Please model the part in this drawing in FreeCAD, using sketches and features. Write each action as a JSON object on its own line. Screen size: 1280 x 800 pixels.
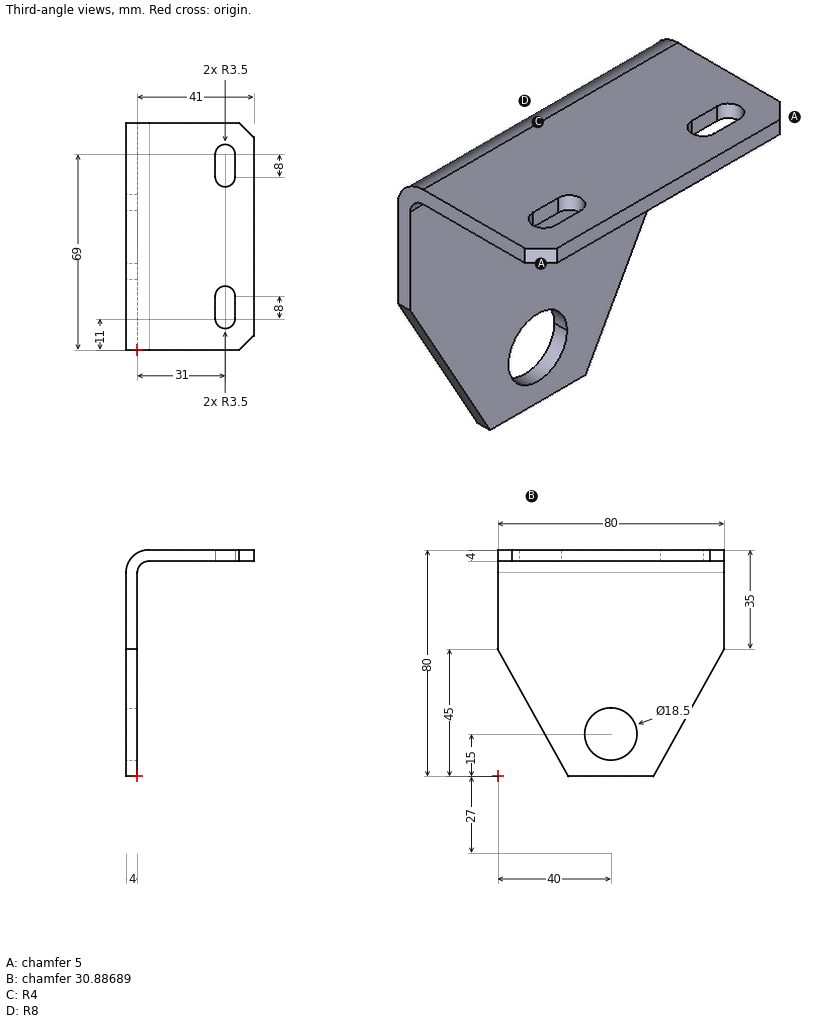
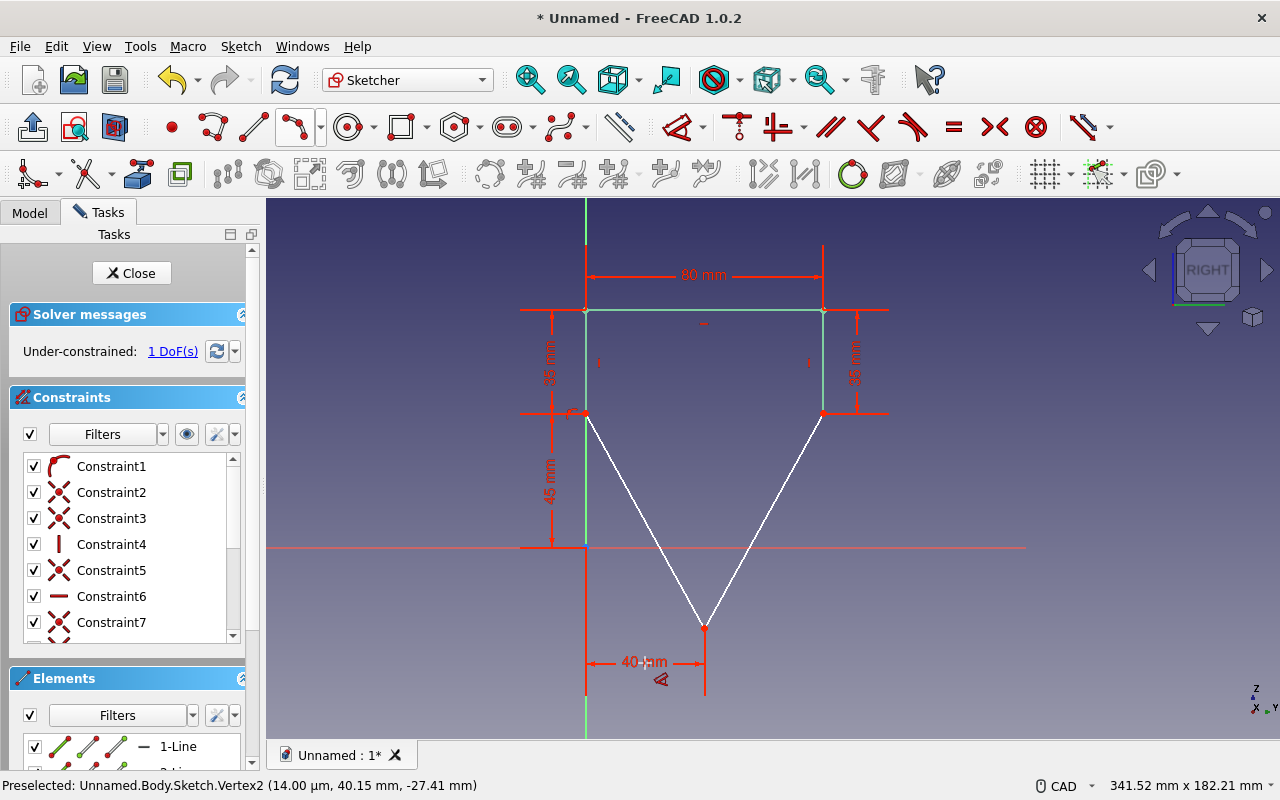
{"action": "left_click", "coordinate": [705, 629]}
{"action": "left_click", "coordinate": [552, 588]}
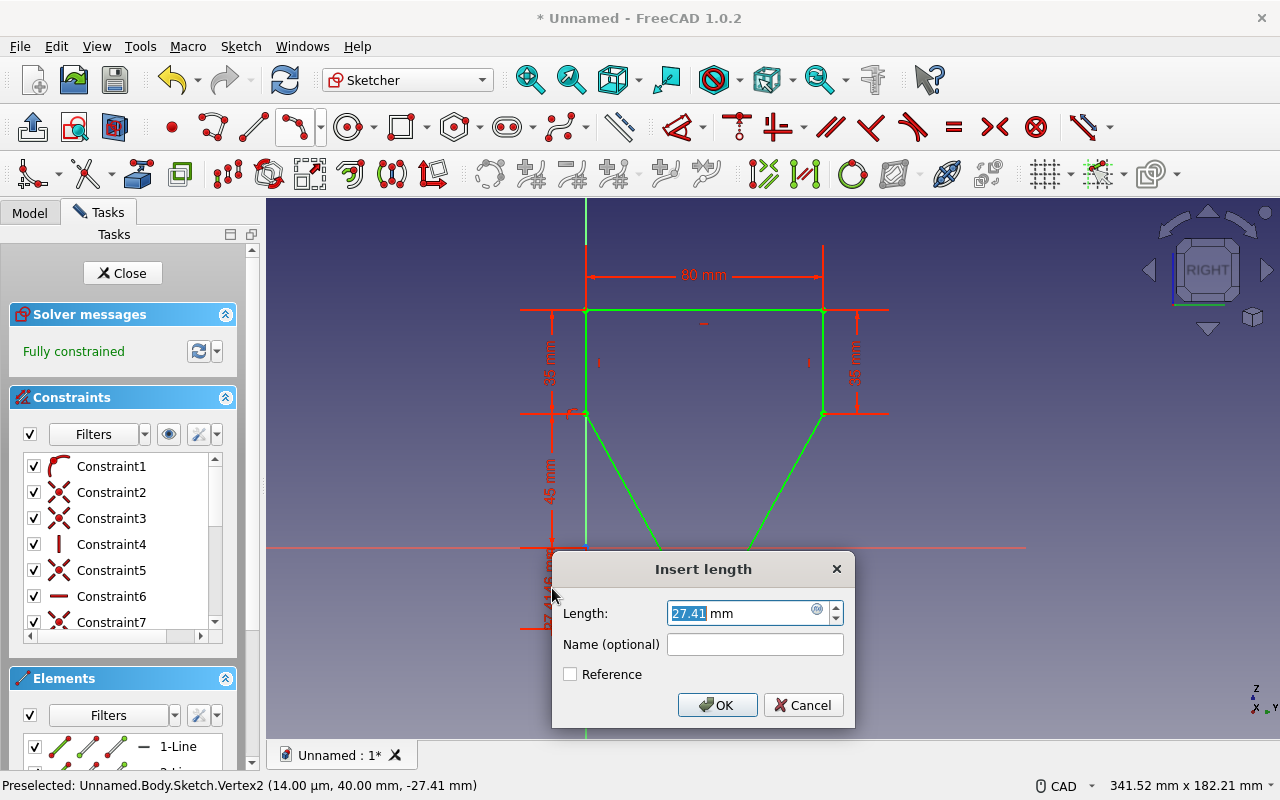
{"action": "type", "text": "27"}
{"action": "key", "text": "Return"}
{"action": "key", "text": "Escape"}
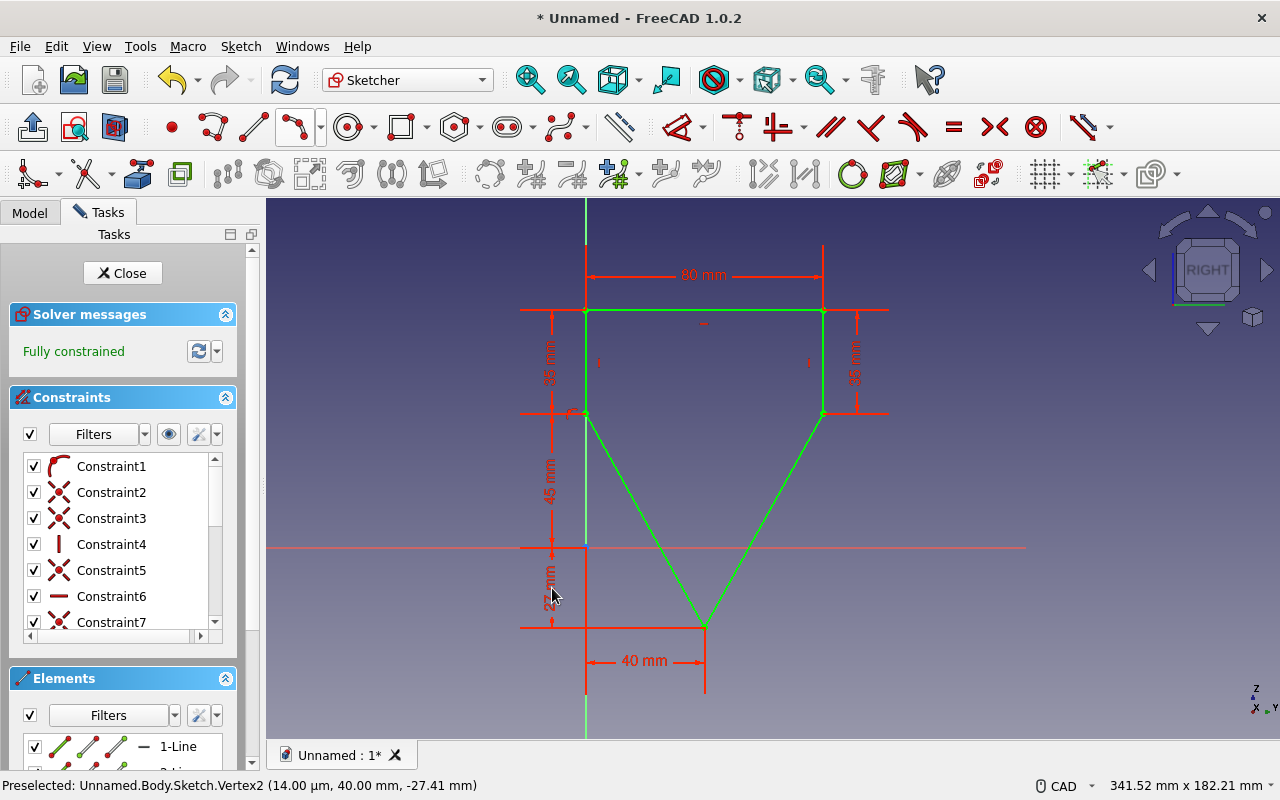
{"action": "left_click", "coordinate": [123, 273]}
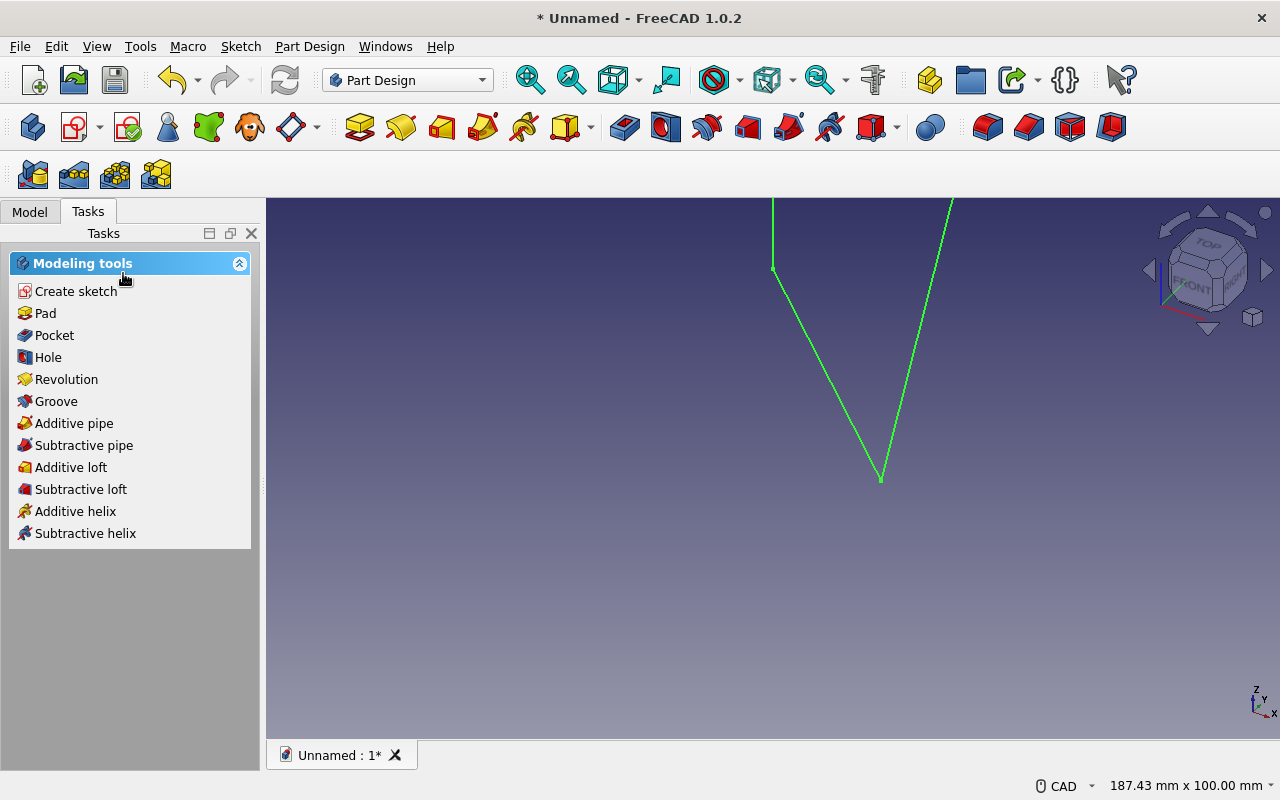
{"action": "left_click", "coordinate": [360, 128]}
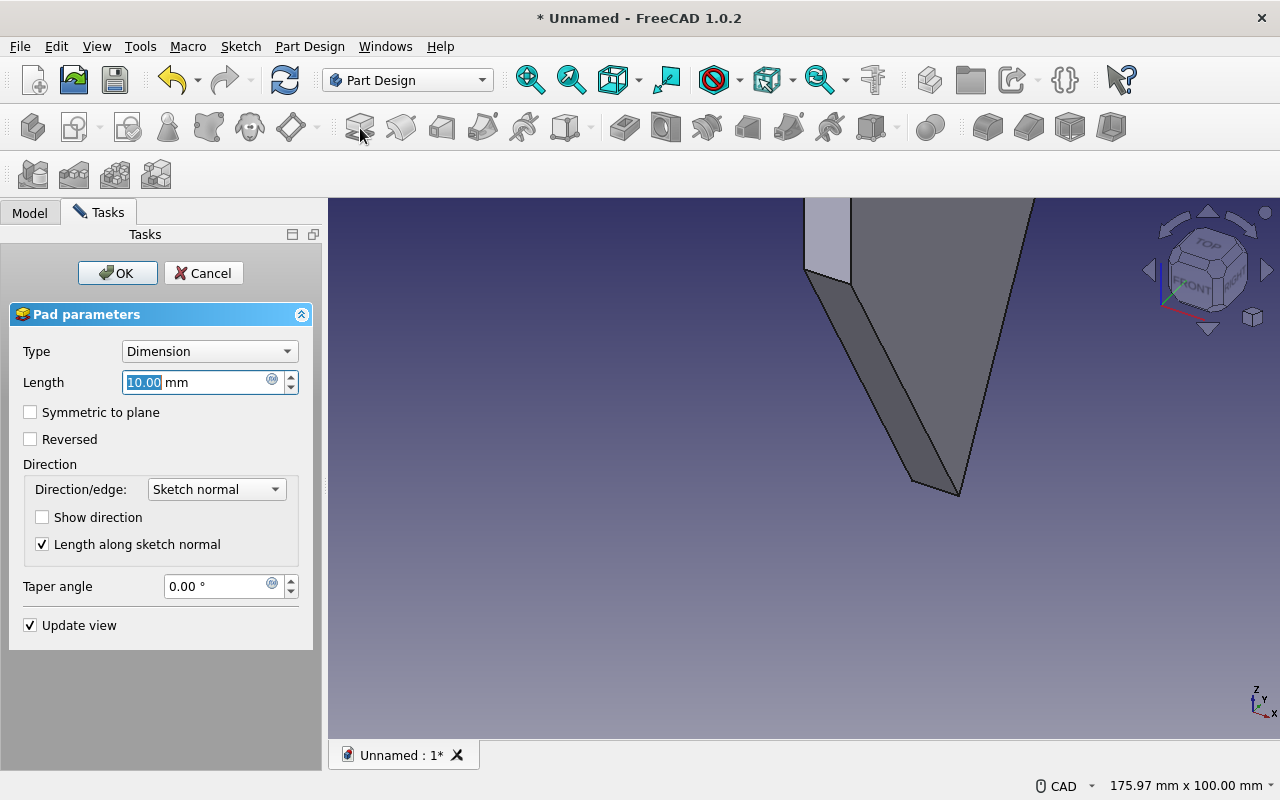
{"action": "type", "text": "4"}
{"action": "key", "text": "Tab"}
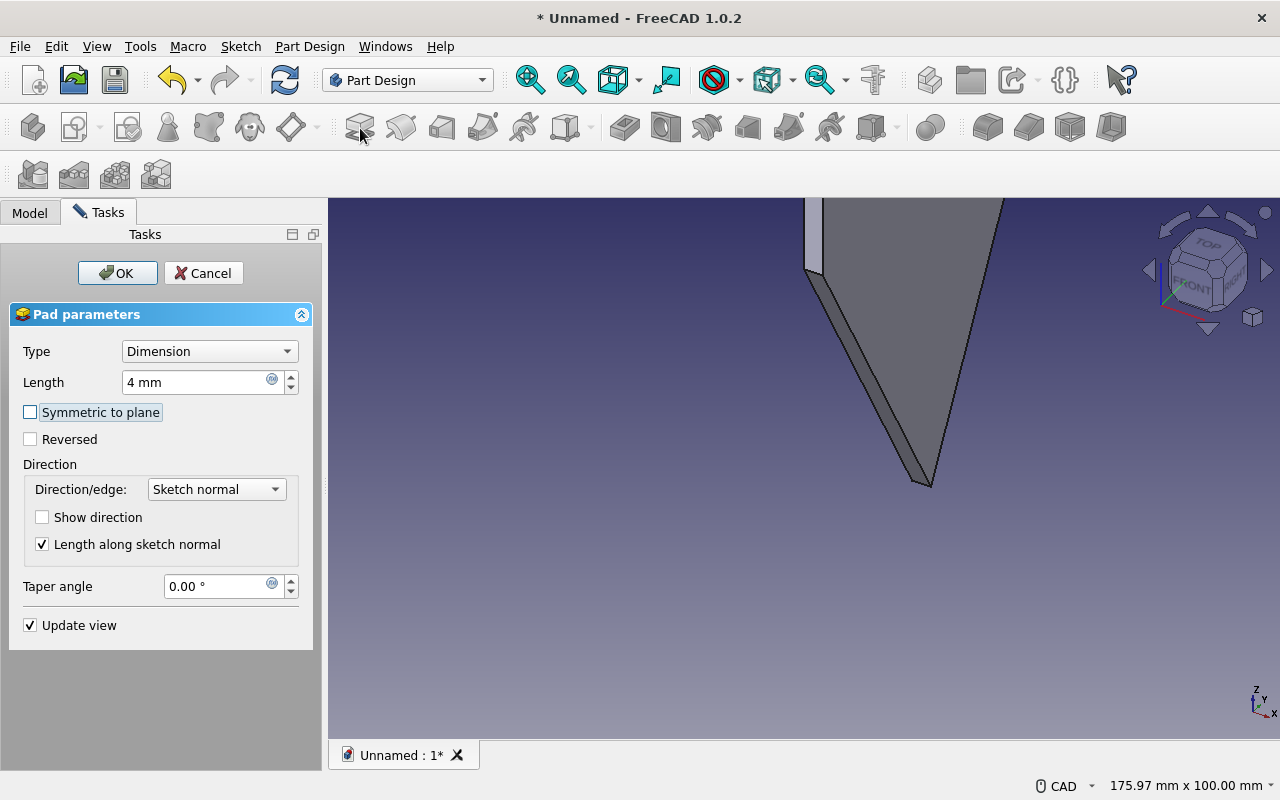
{"action": "left_click", "coordinate": [31, 439]}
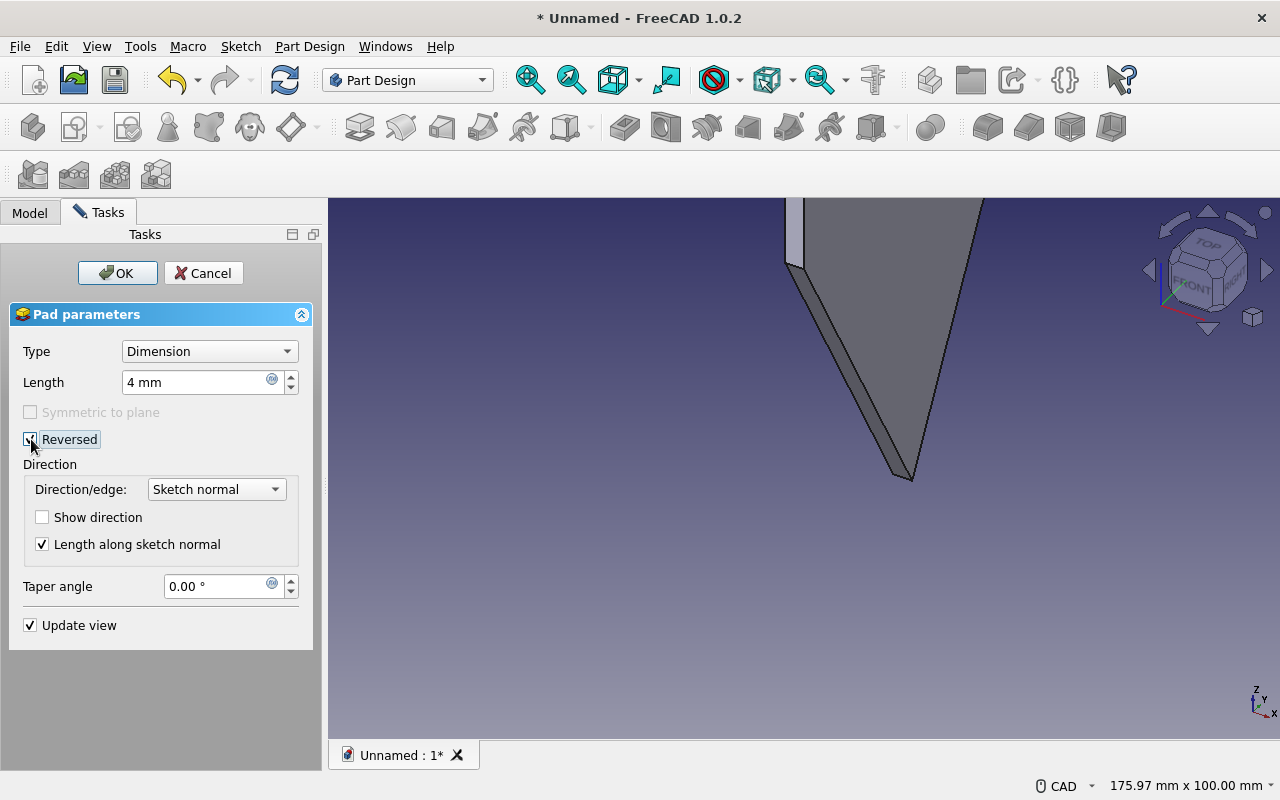
{"action": "left_click", "coordinate": [118, 273]}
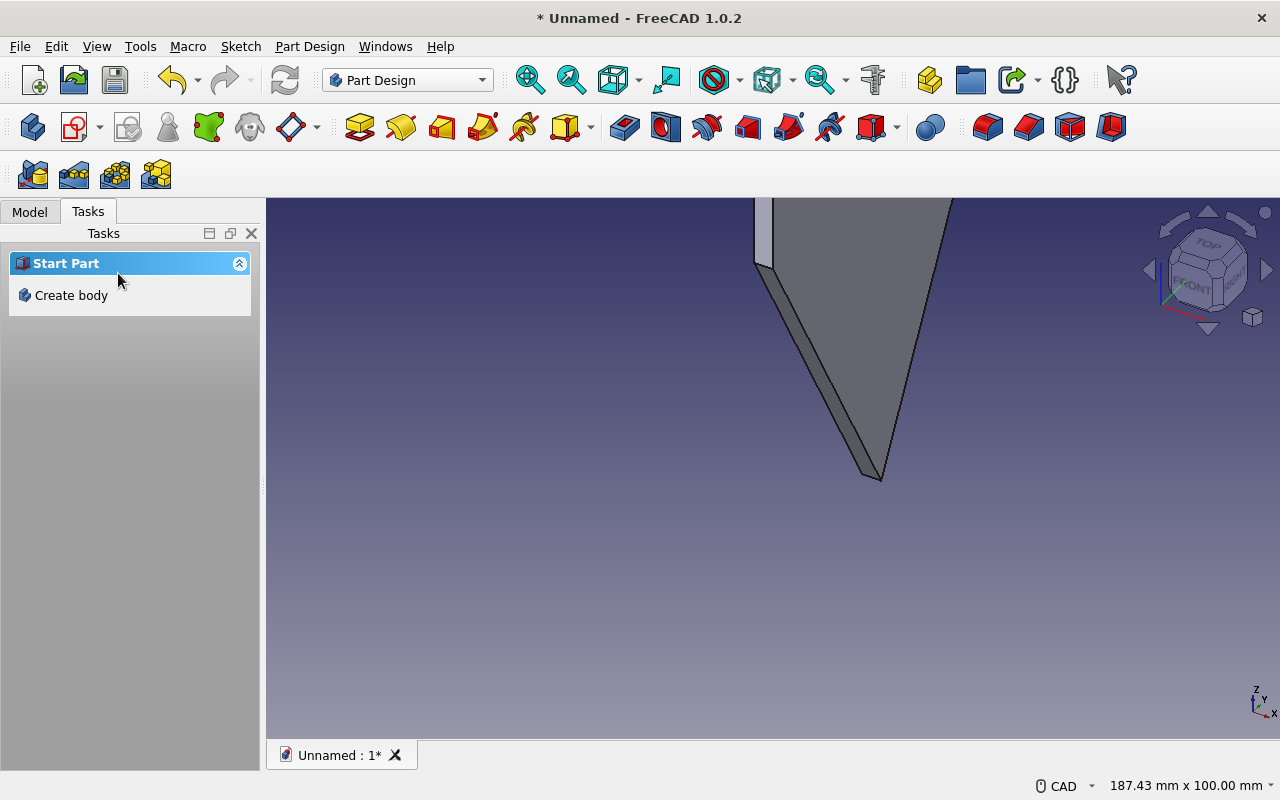
{"action": "key", "text": "v f"}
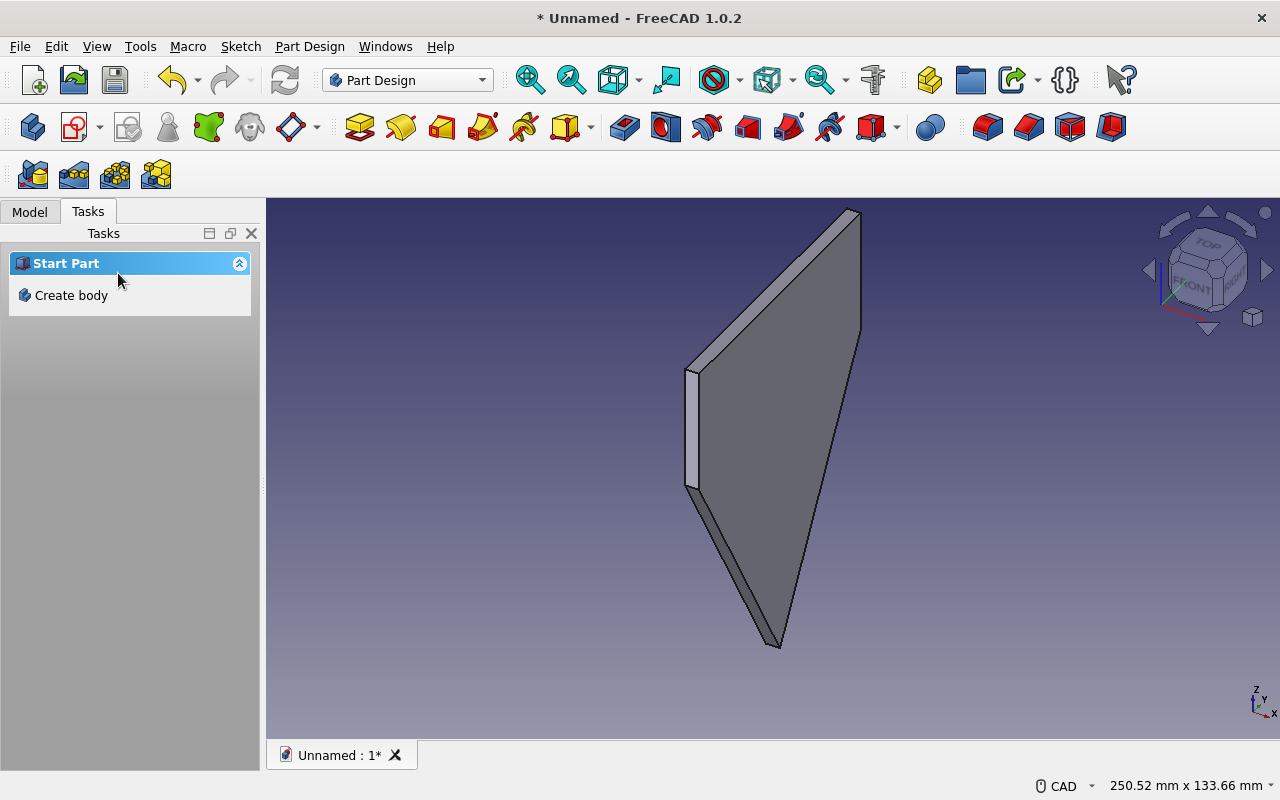
{"action": "left_click", "coordinate": [780, 419]}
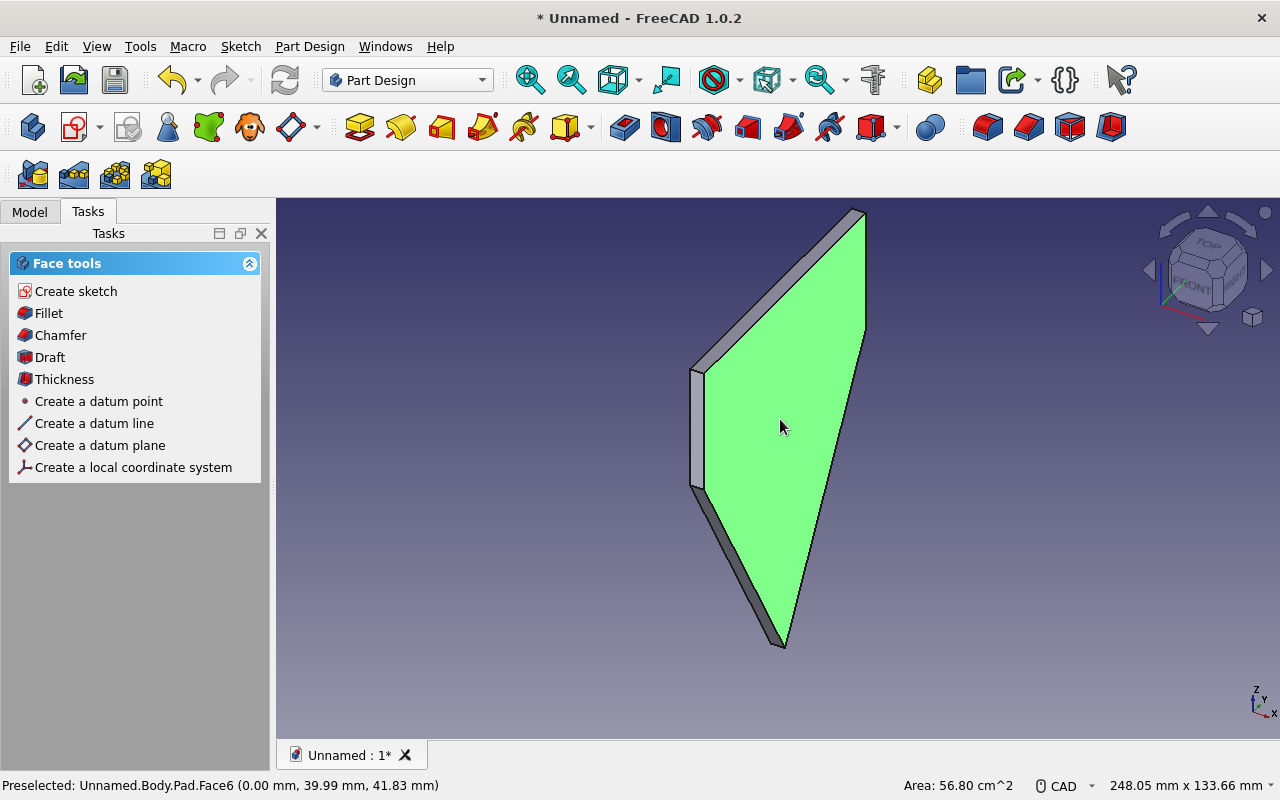
{"action": "left_click", "coordinate": [74, 128]}